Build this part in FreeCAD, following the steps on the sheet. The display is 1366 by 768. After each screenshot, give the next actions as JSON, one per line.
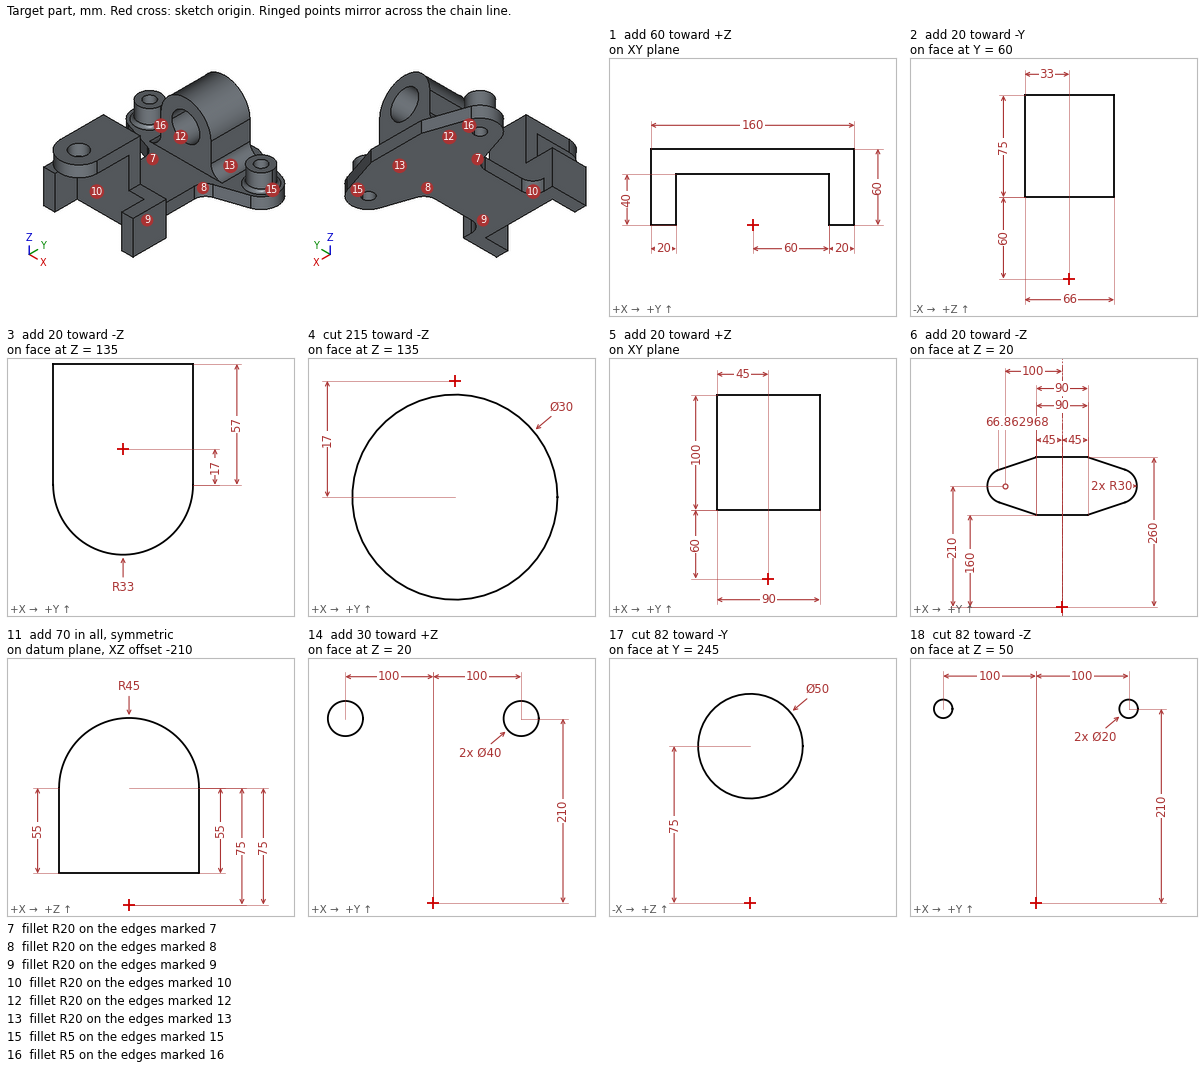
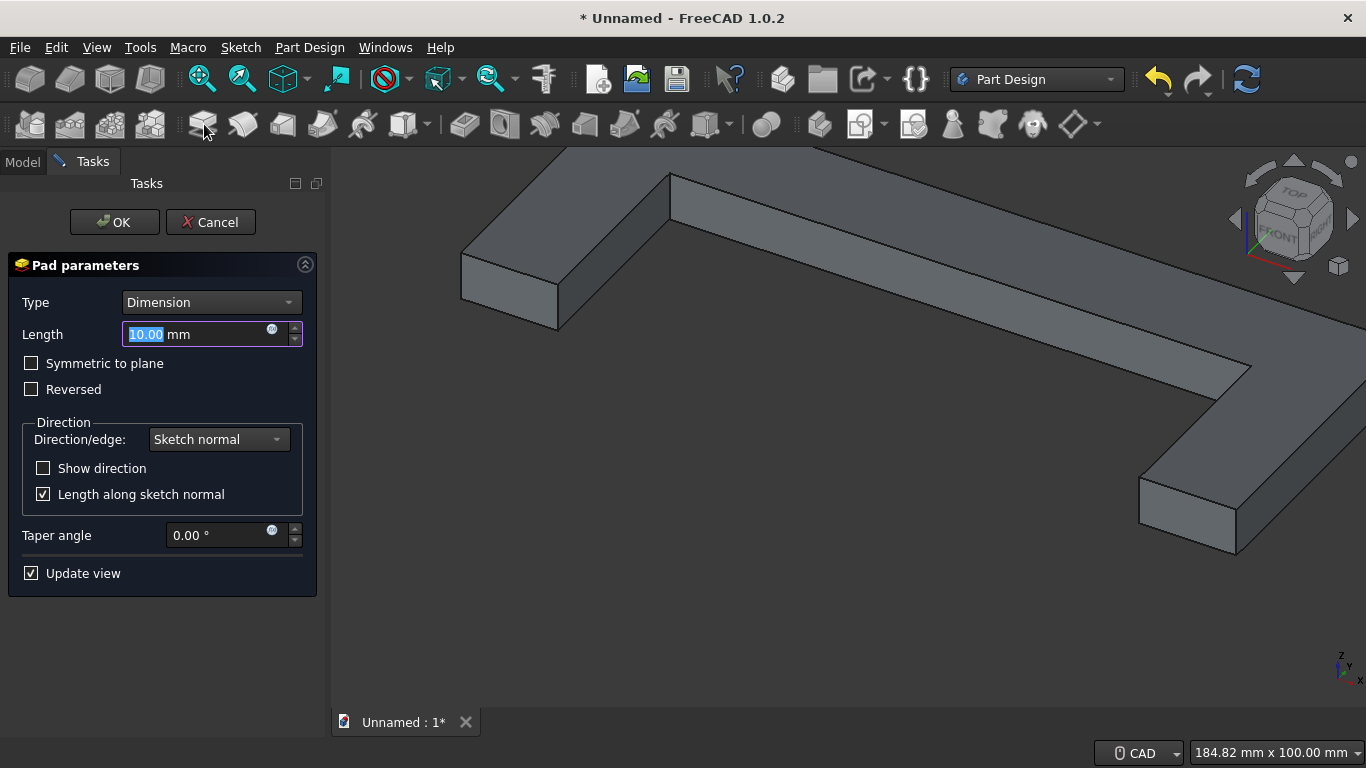
{"action": "type", "text": "60"}
{"action": "key", "text": "Tab"}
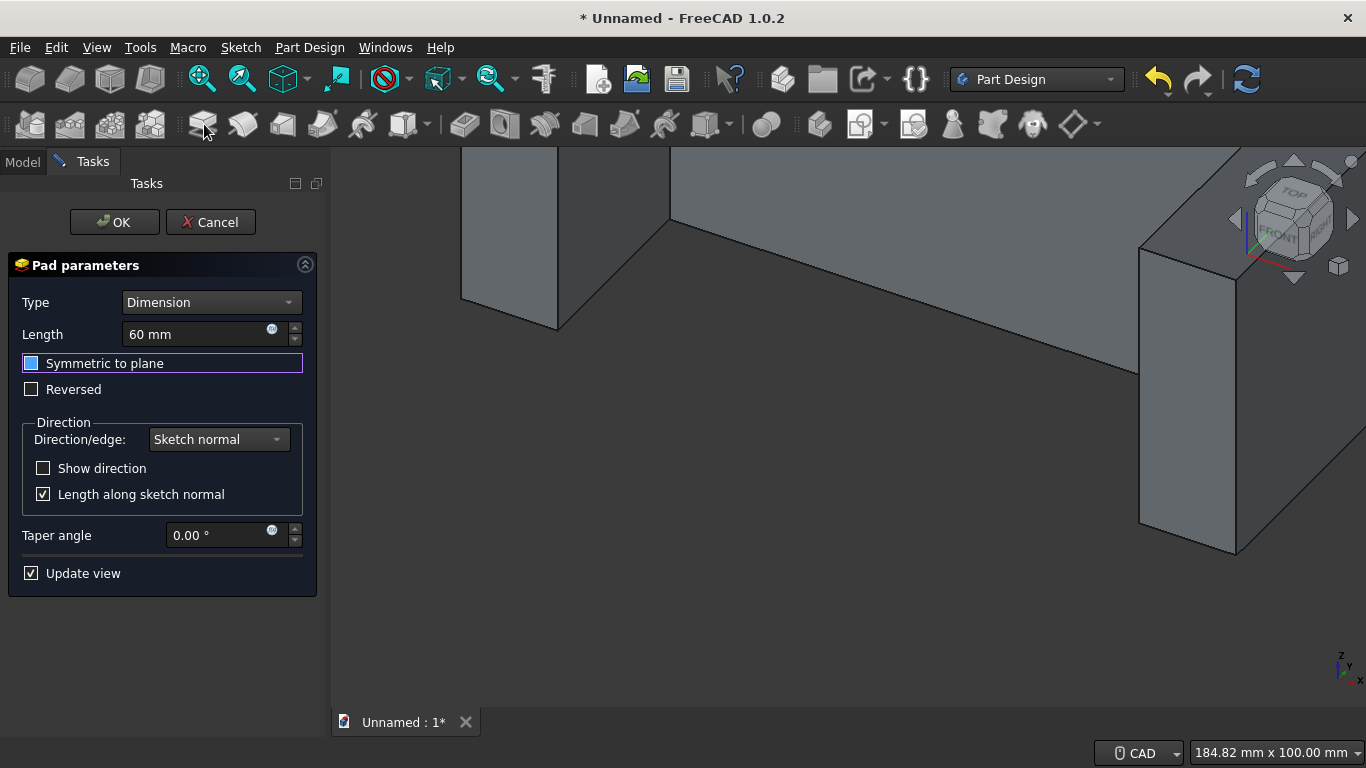
{"action": "left_click", "coordinate": [115, 222]}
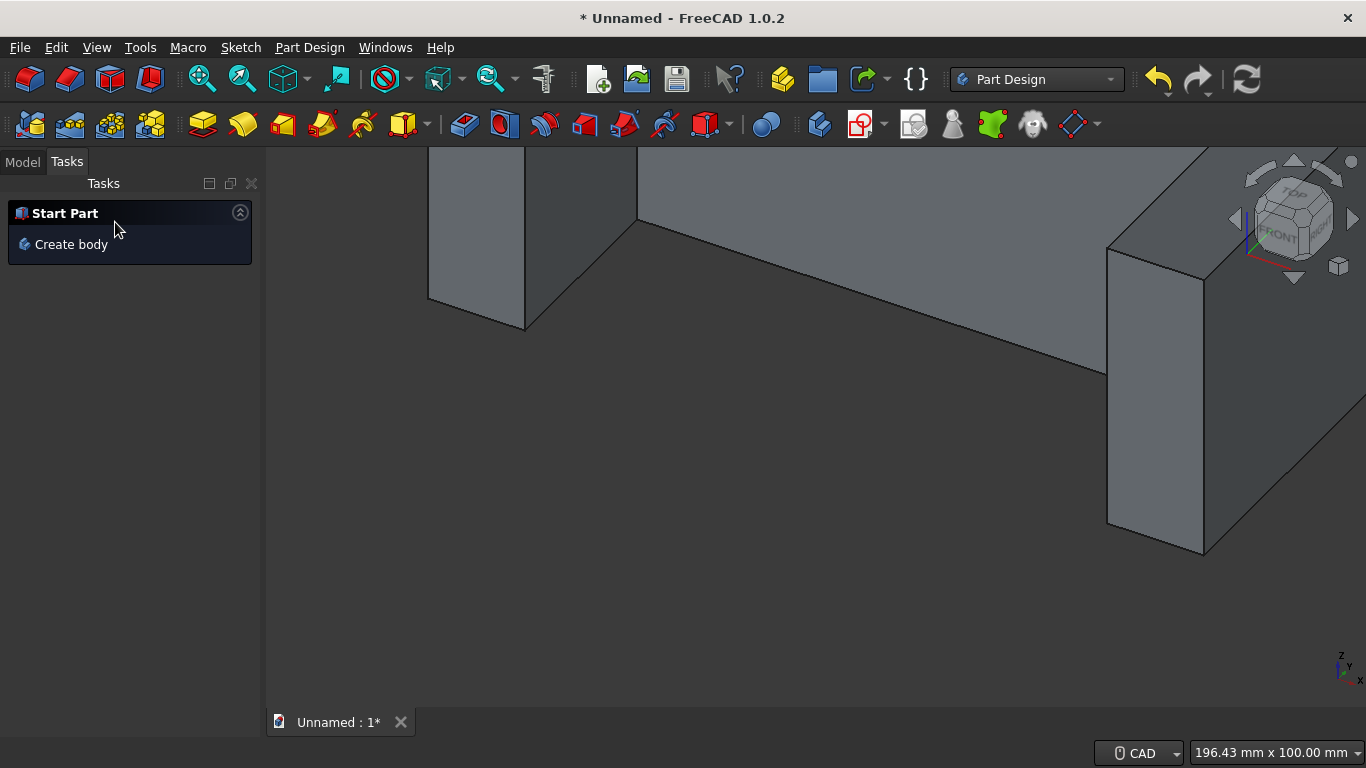
{"action": "key", "text": "v f"}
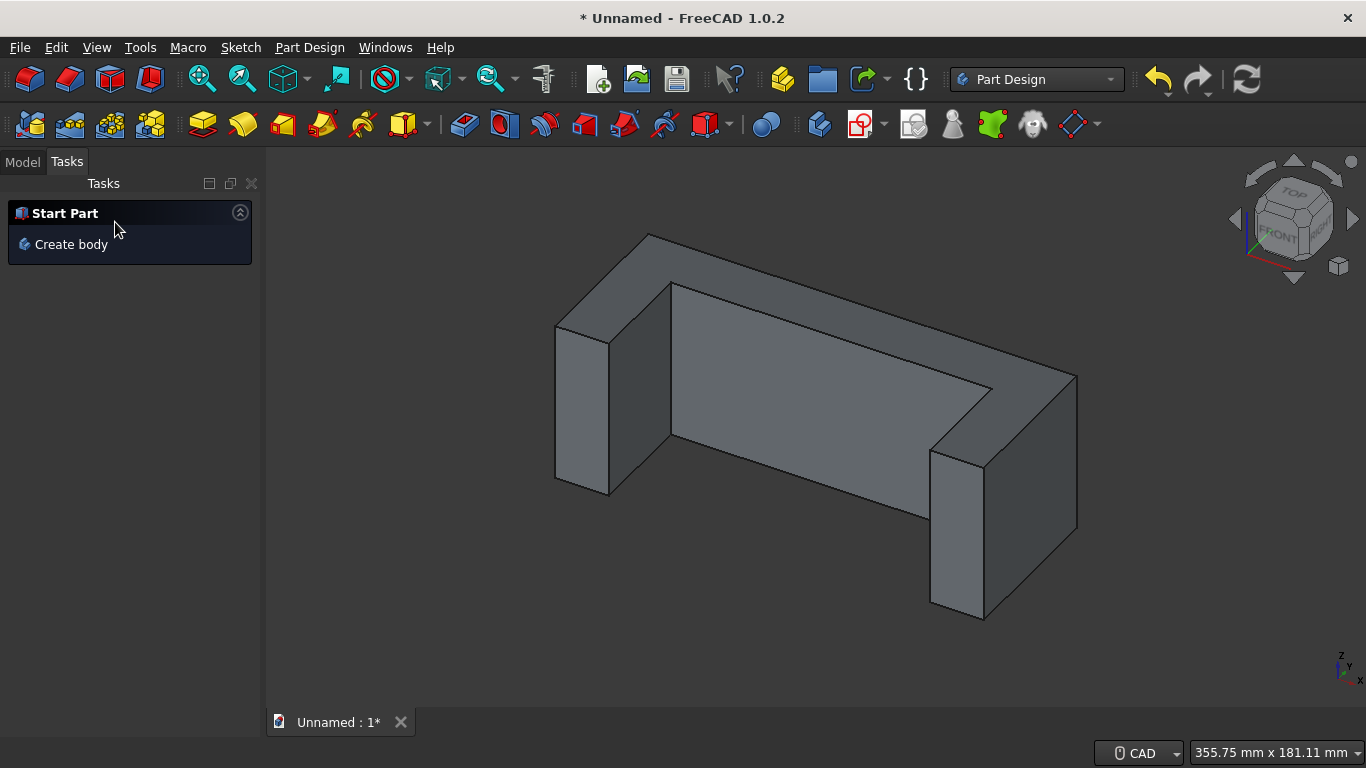
{"action": "key", "text": "4"}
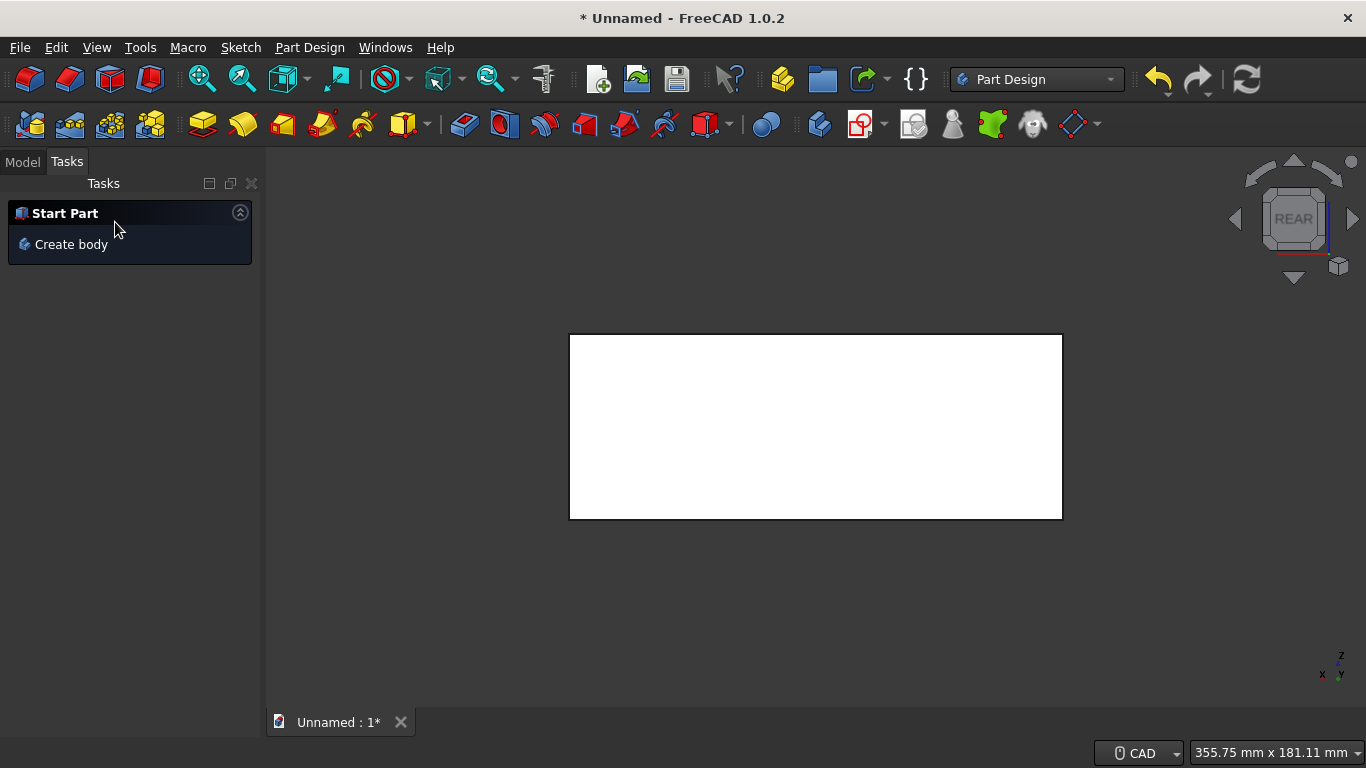
{"action": "key", "text": "v f"}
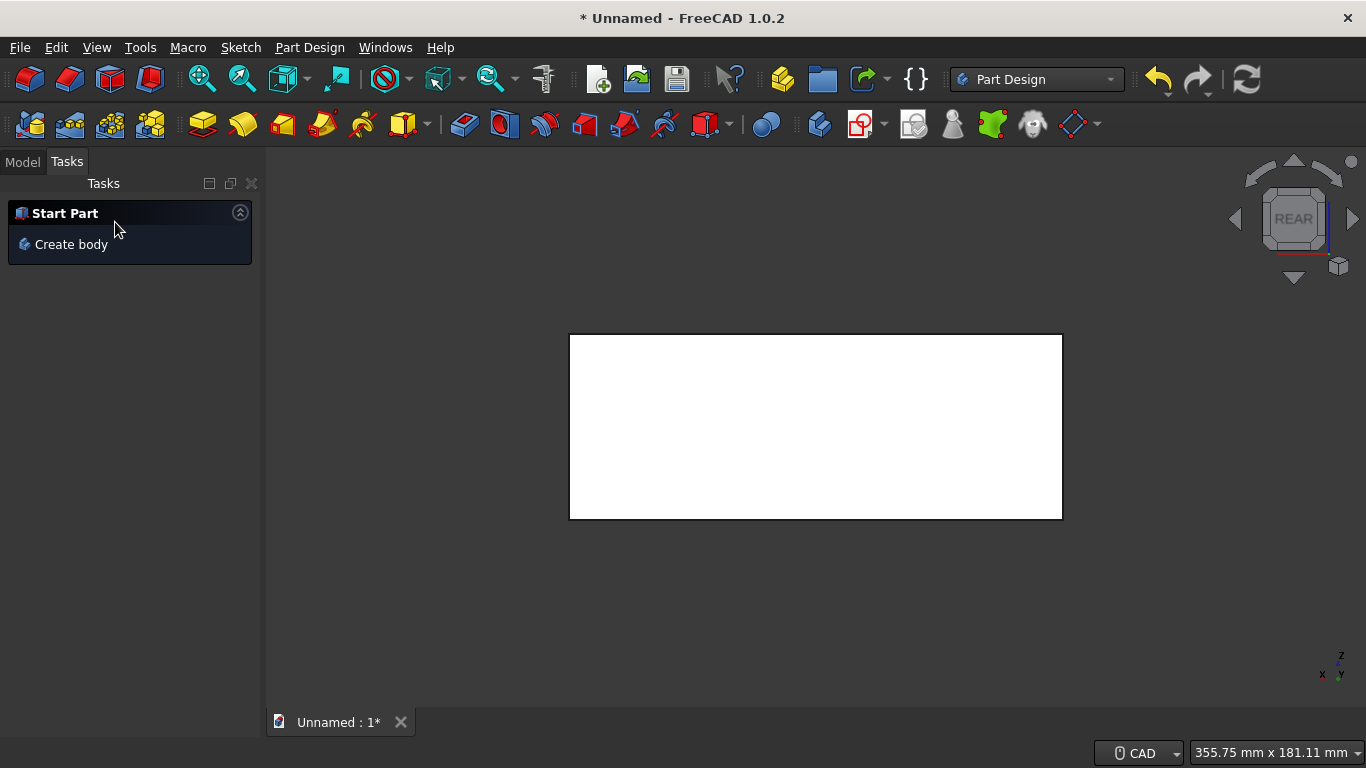
{"action": "left_click", "coordinate": [675, 426]}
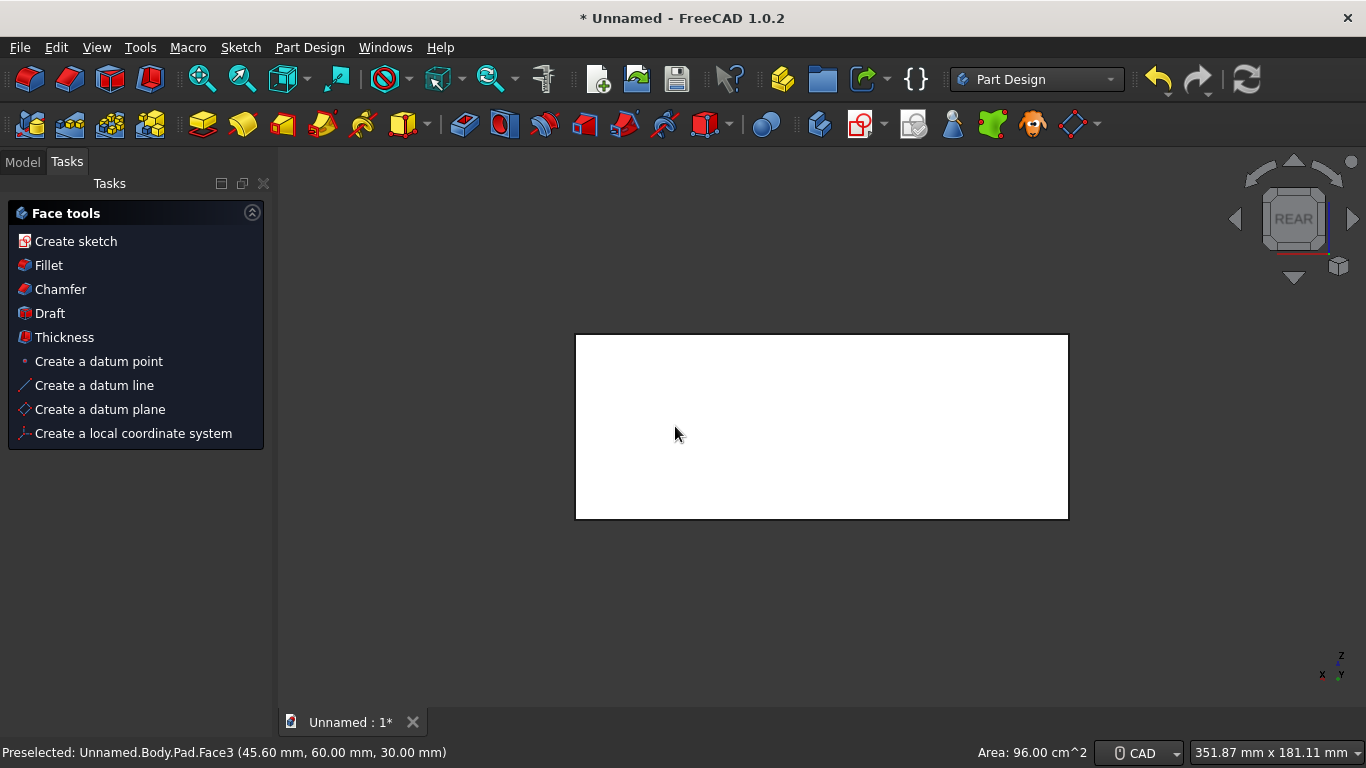
{"action": "left_click", "coordinate": [860, 124]}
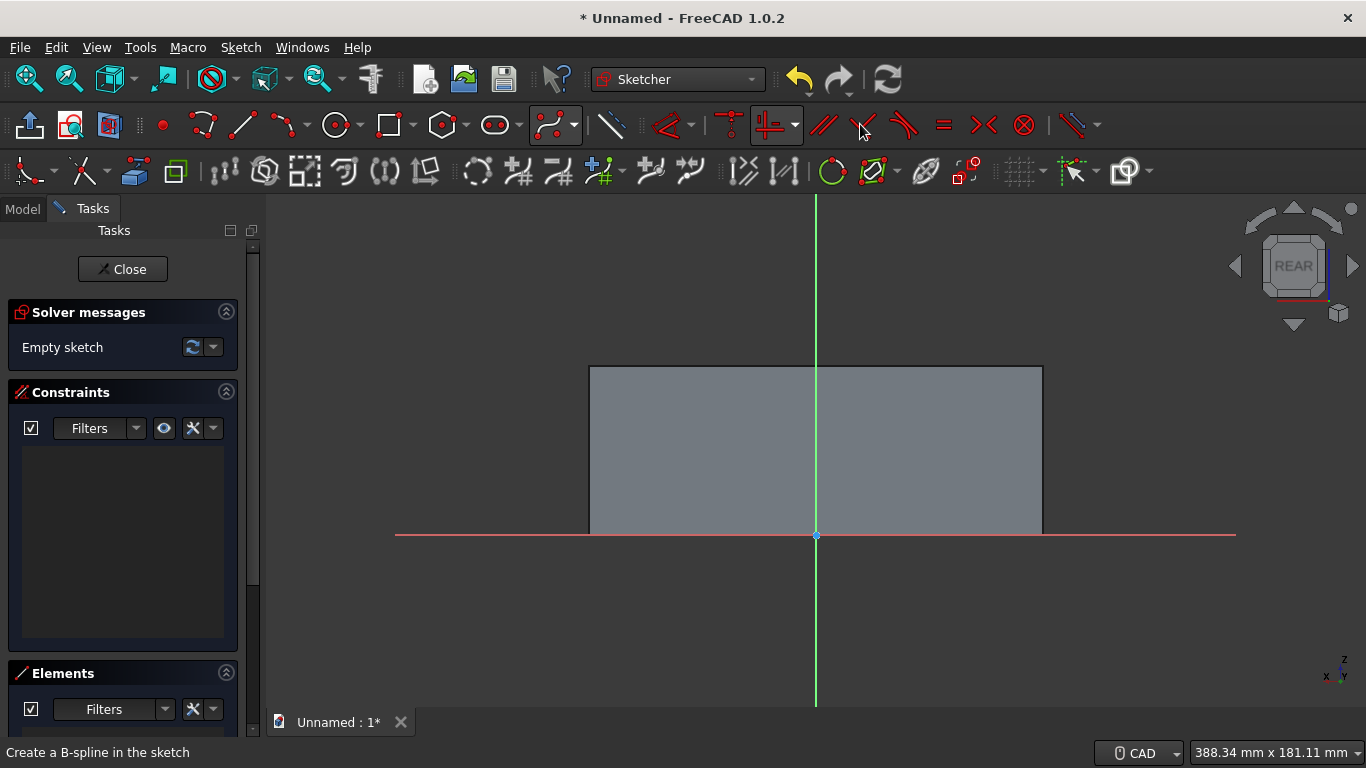
{"action": "scroll", "coordinate": [438, 679], "scroll_direction": "down", "scroll_amount": 1}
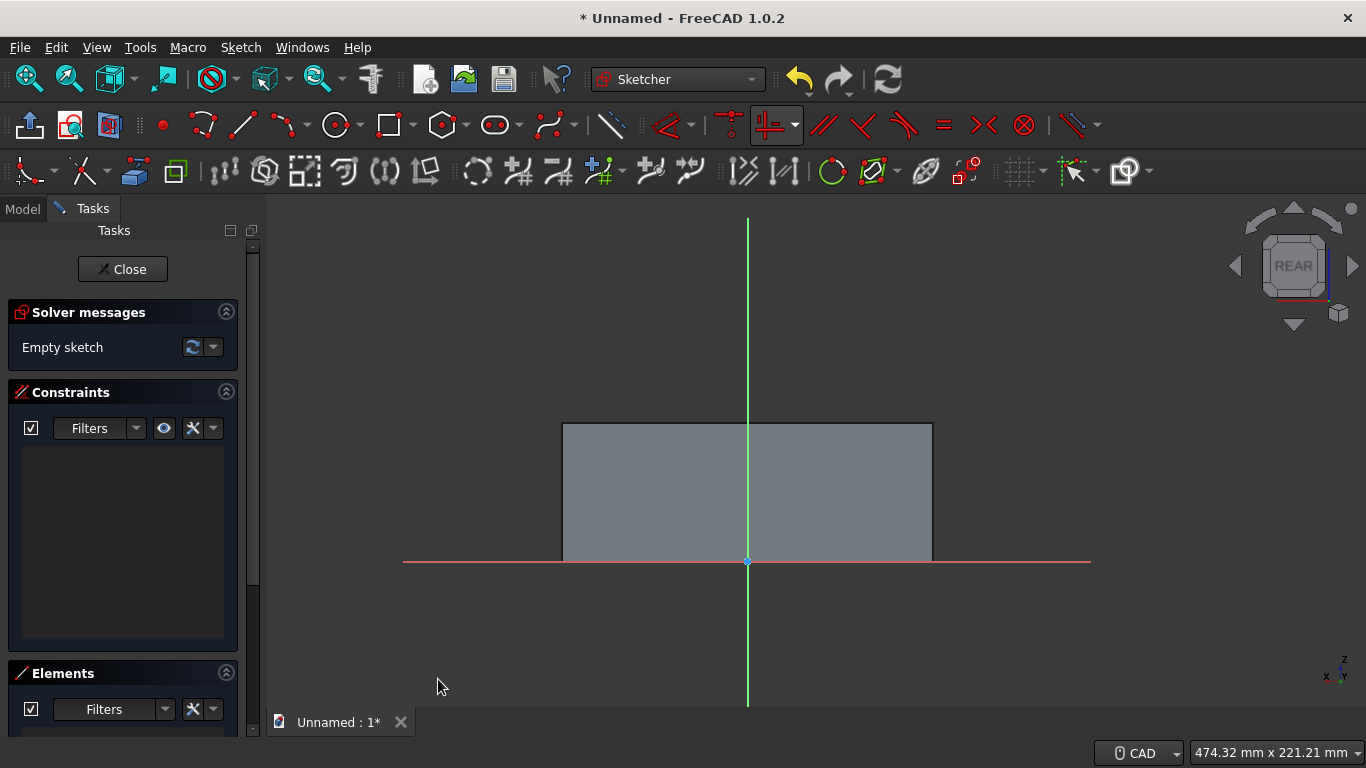
{"action": "key", "text": "g r"}